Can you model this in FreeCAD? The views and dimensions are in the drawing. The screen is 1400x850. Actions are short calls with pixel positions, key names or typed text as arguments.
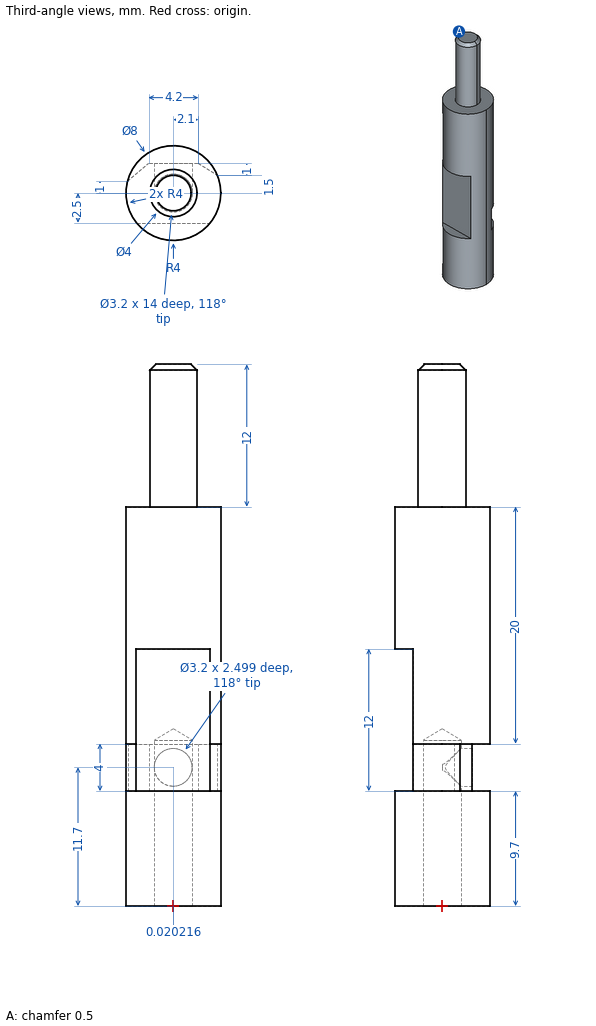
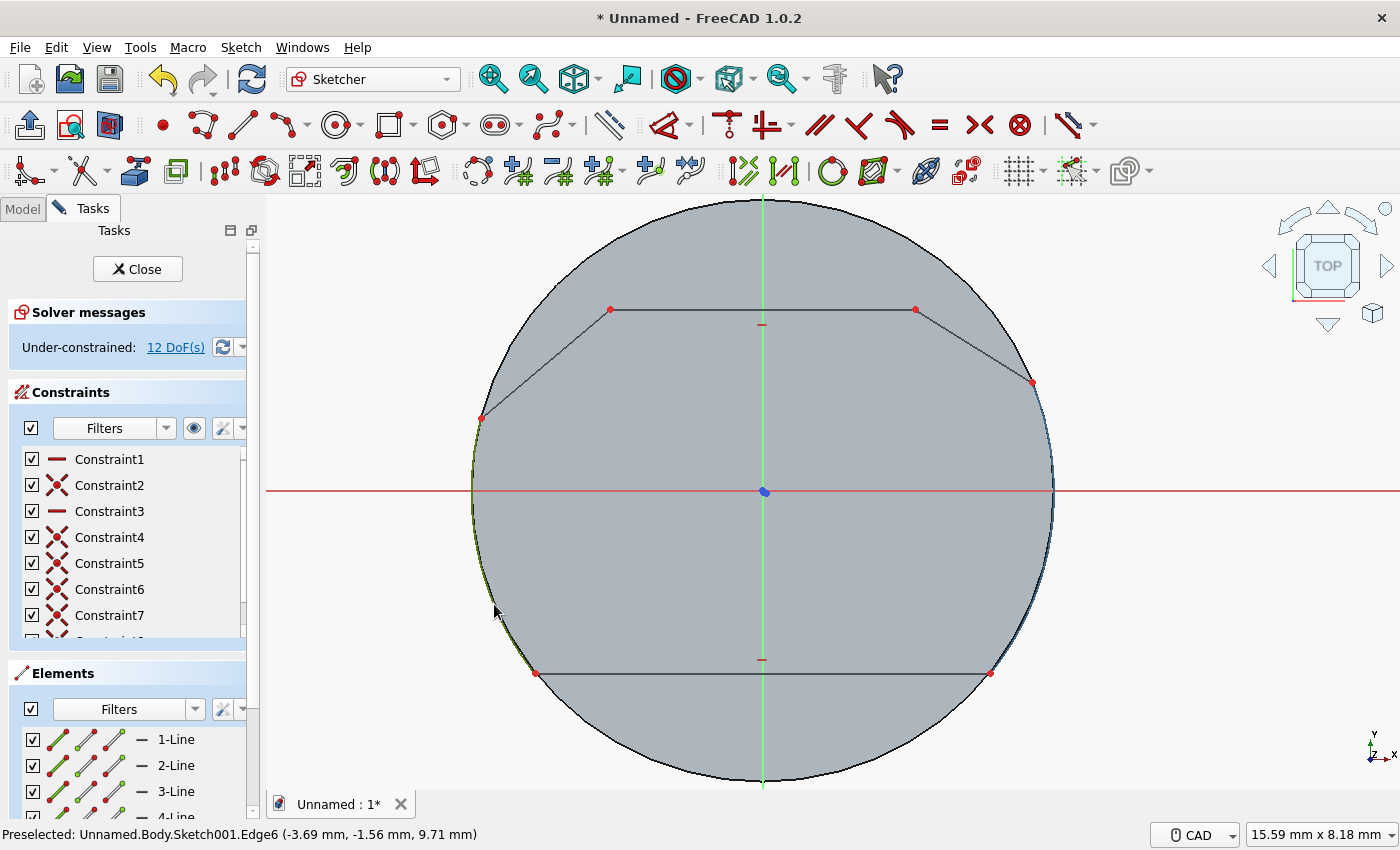
key(c)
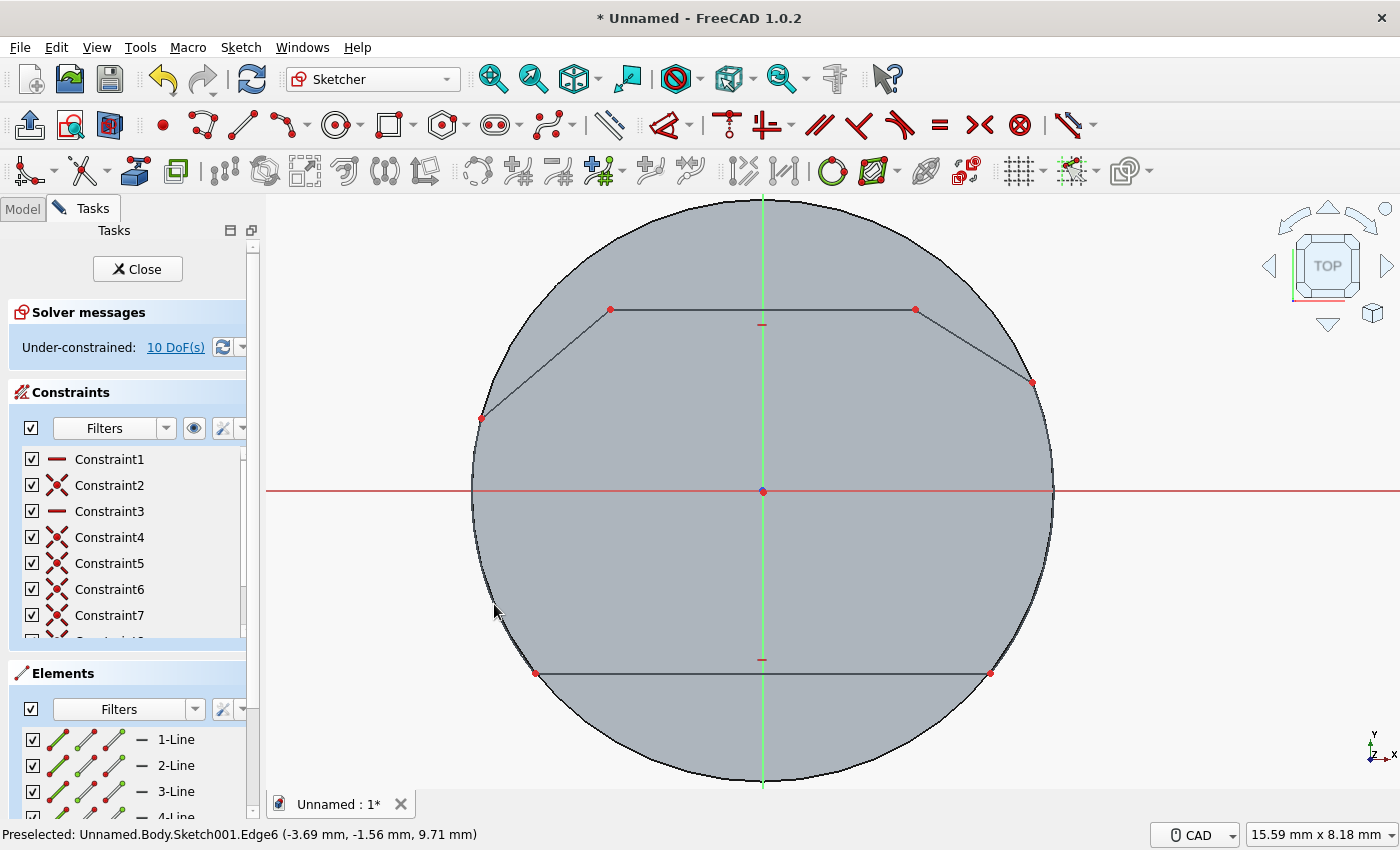
drag(753, 481, 774, 503)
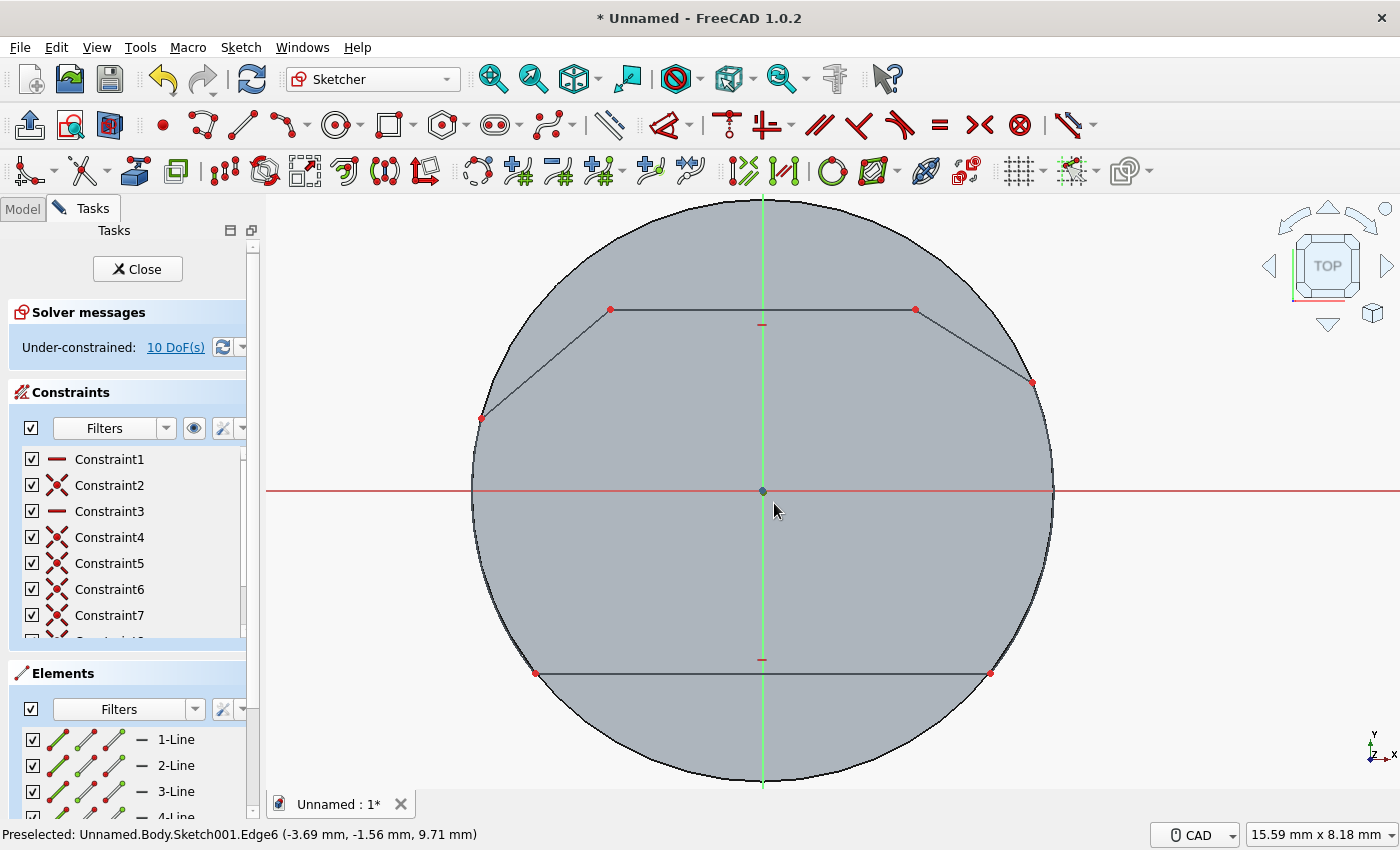
key(c)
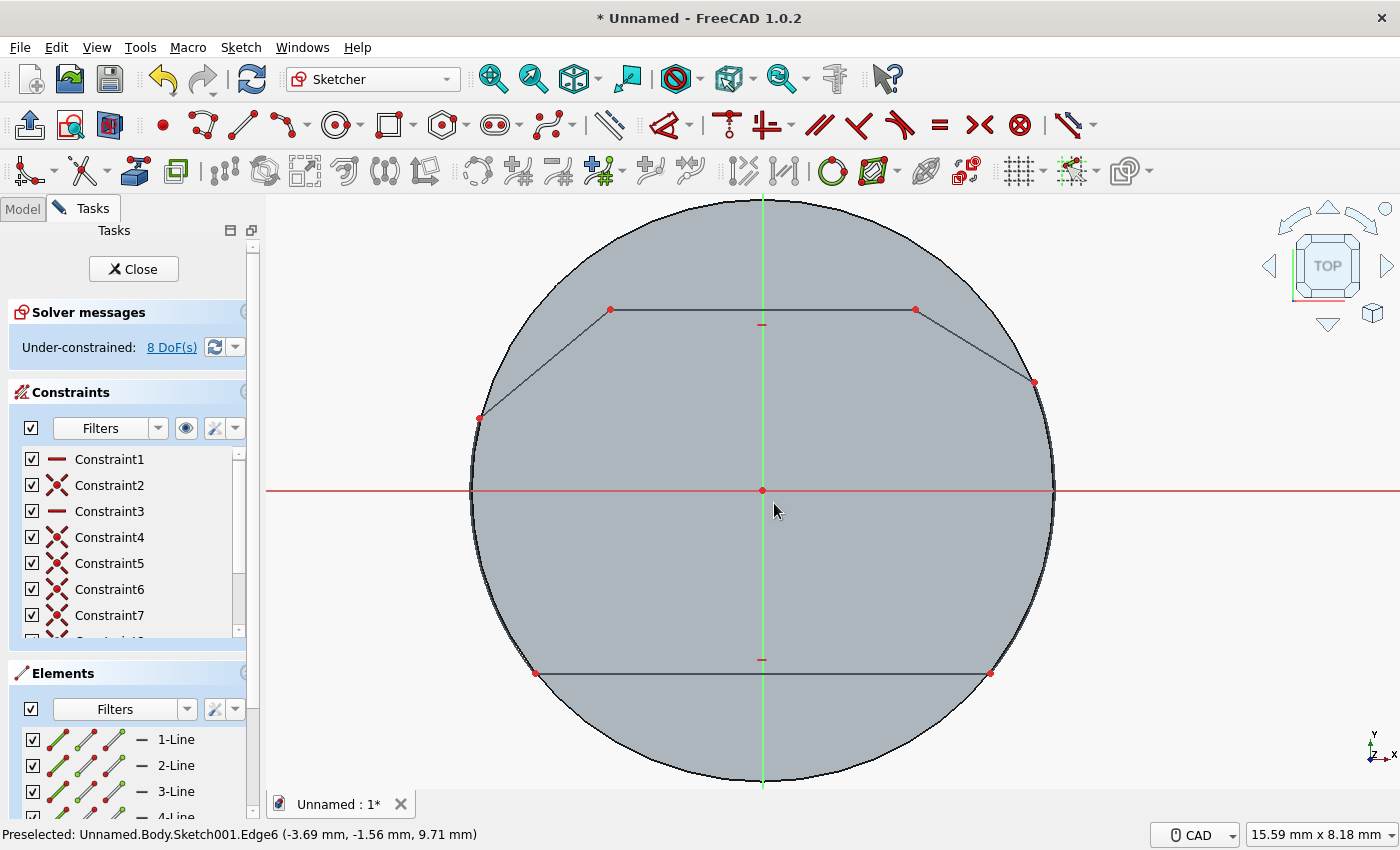
click(1036, 594)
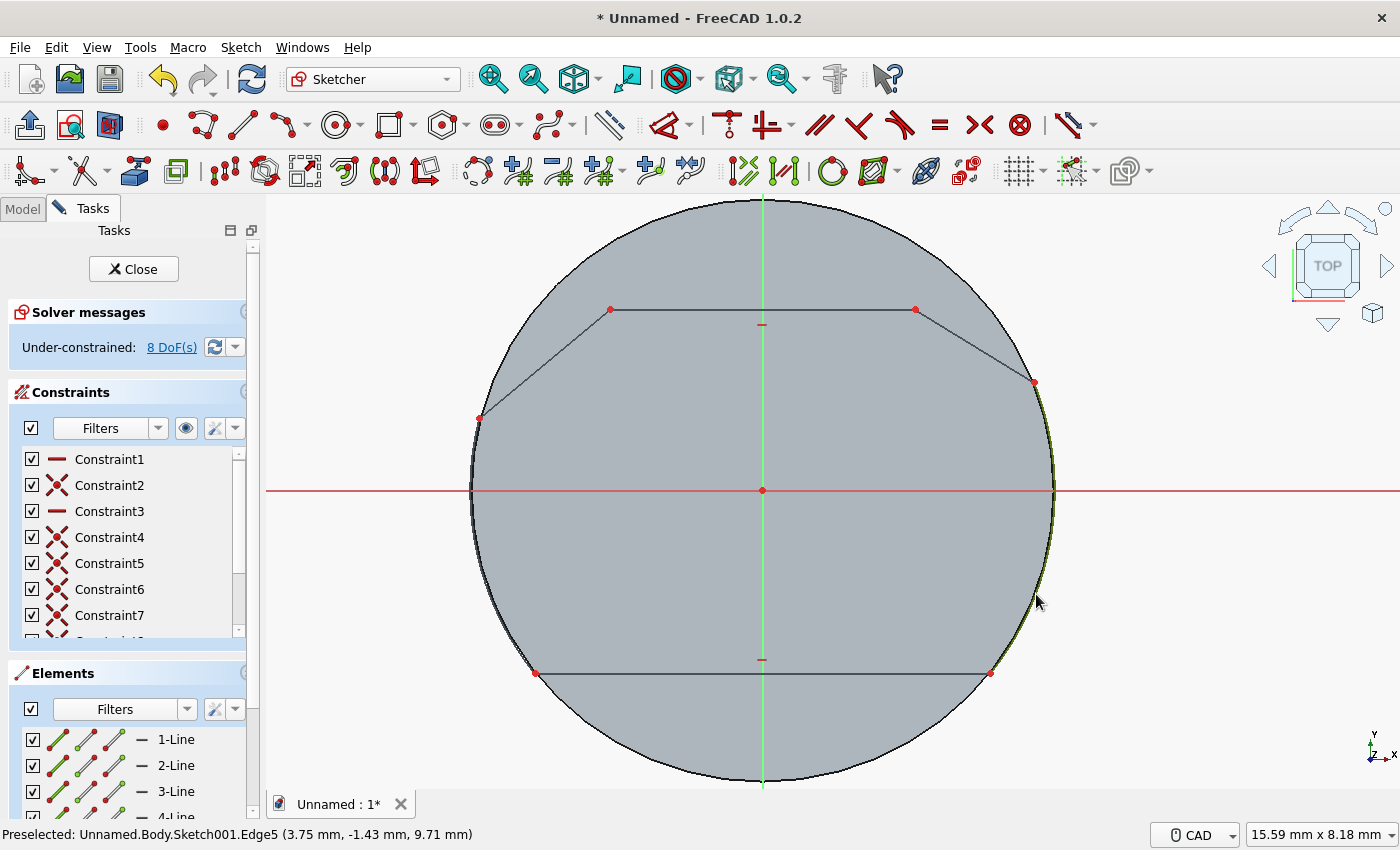
click(493, 605)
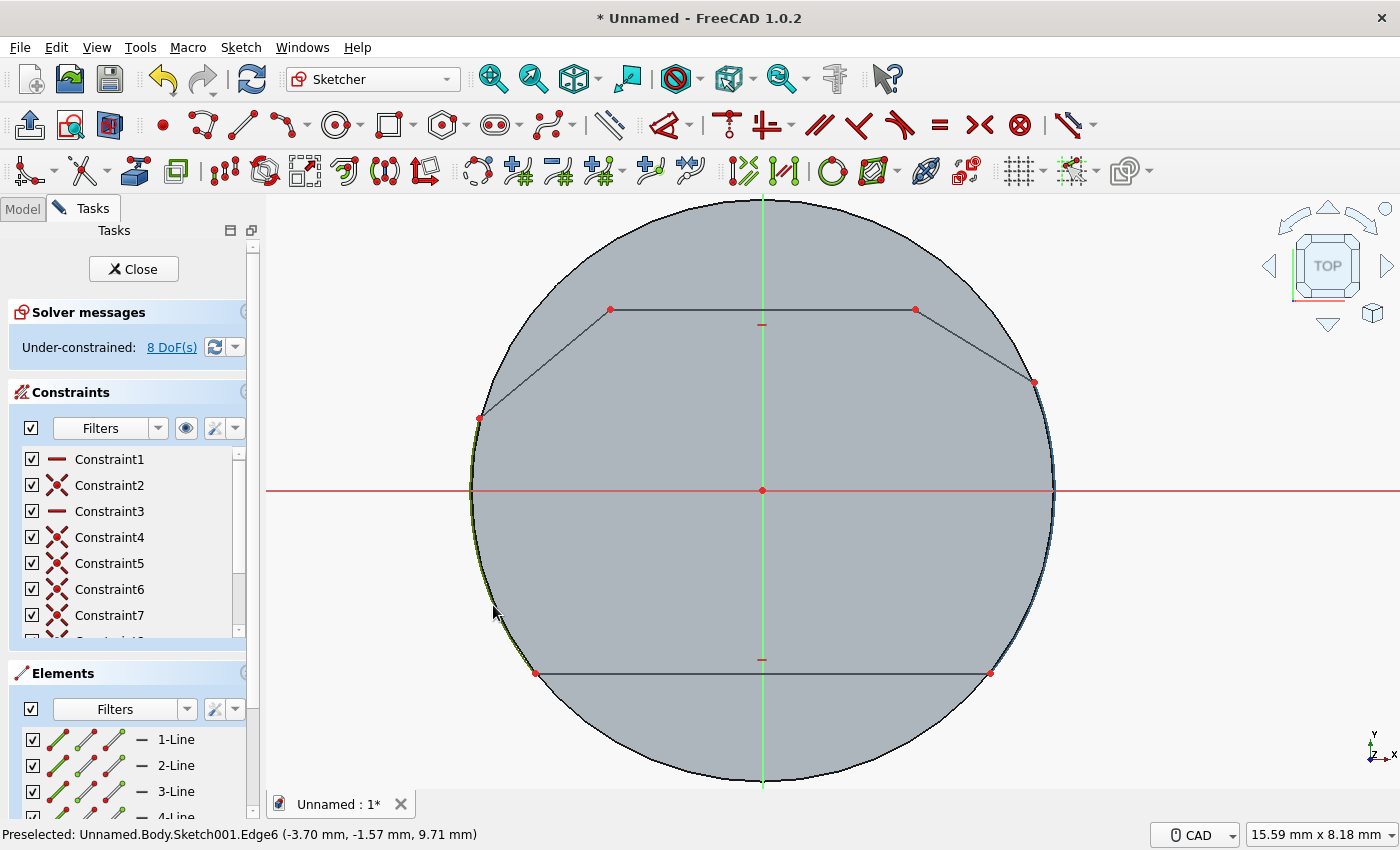
key(e)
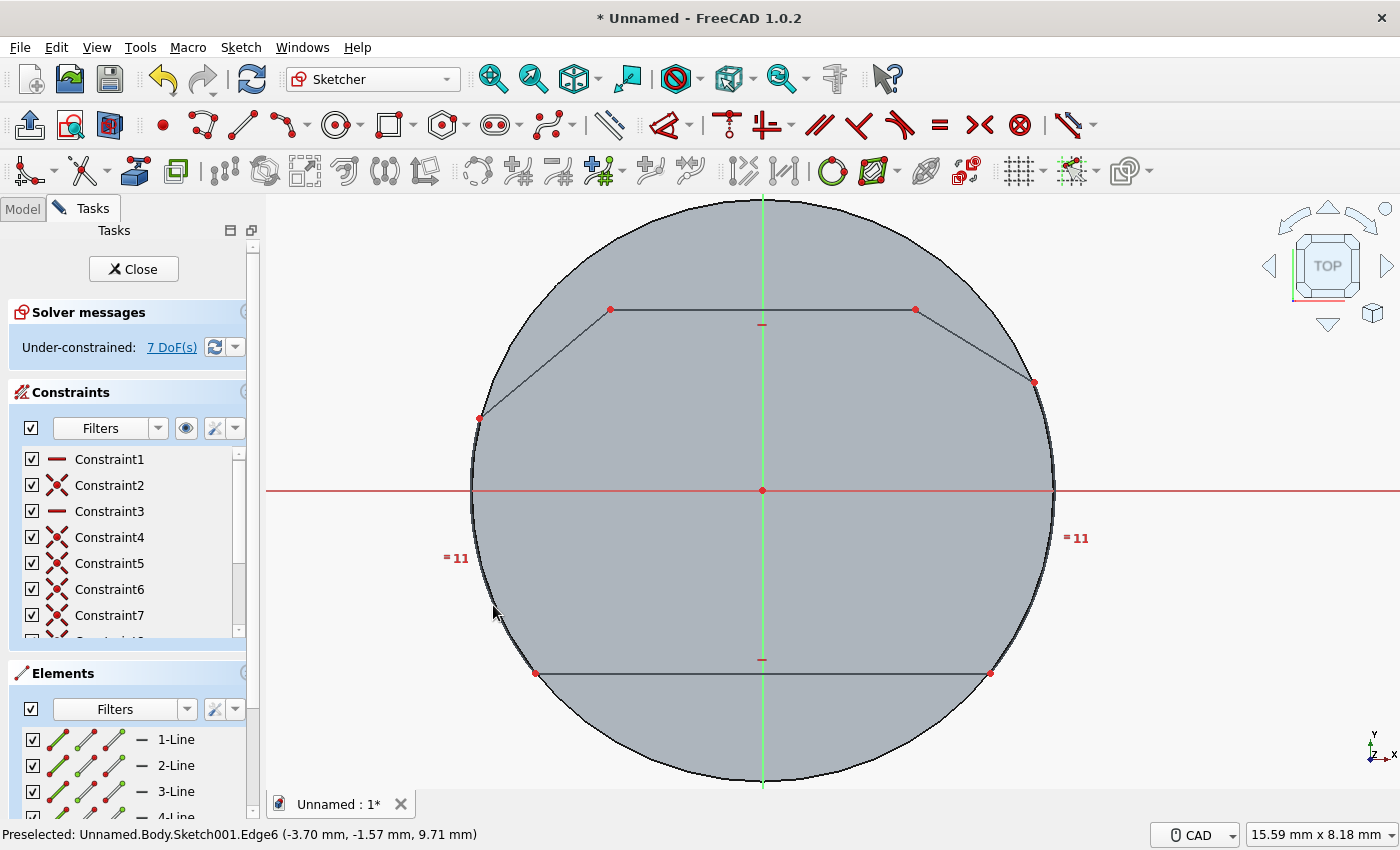
key(d)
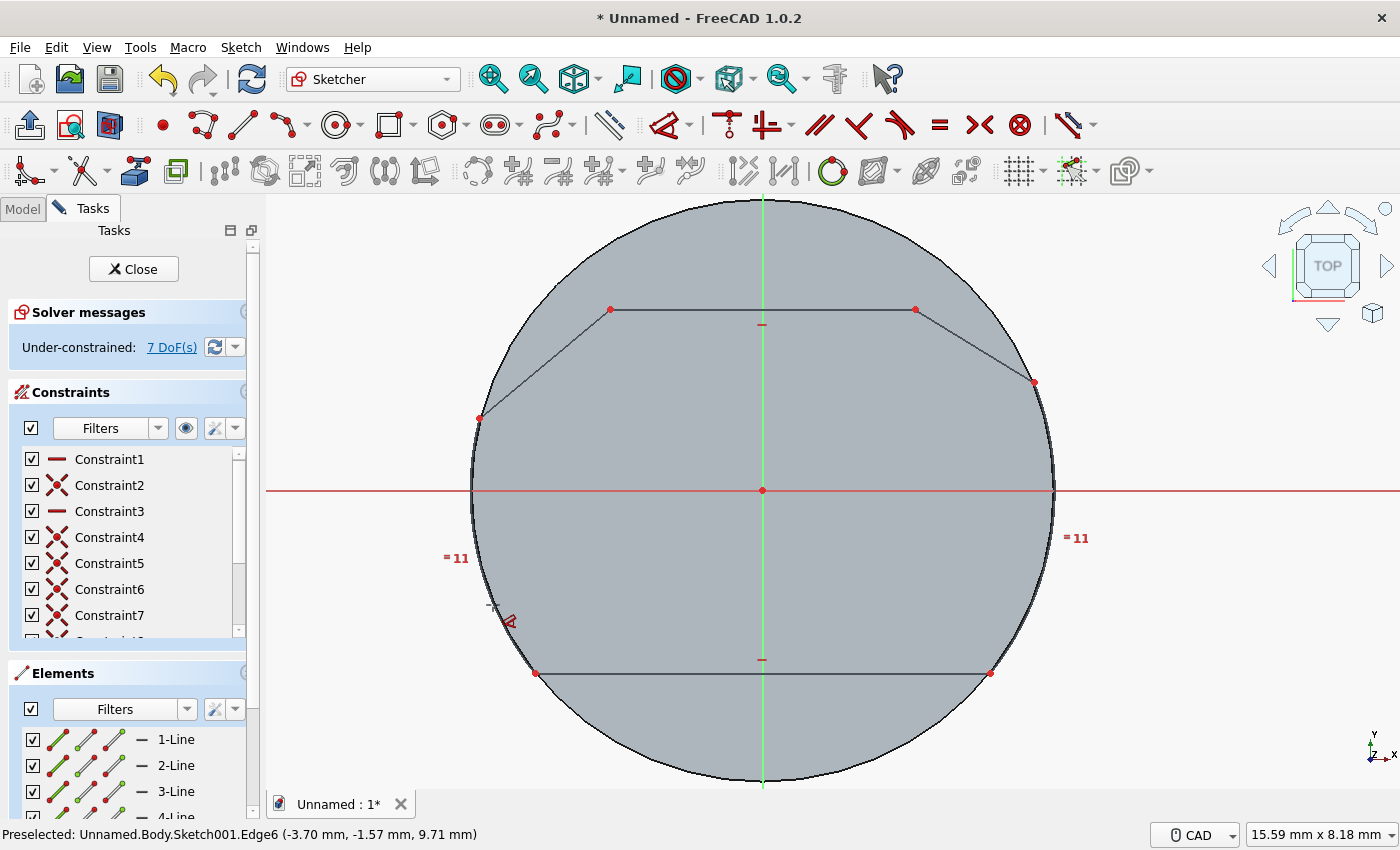
click(1036, 594)
click(1066, 605)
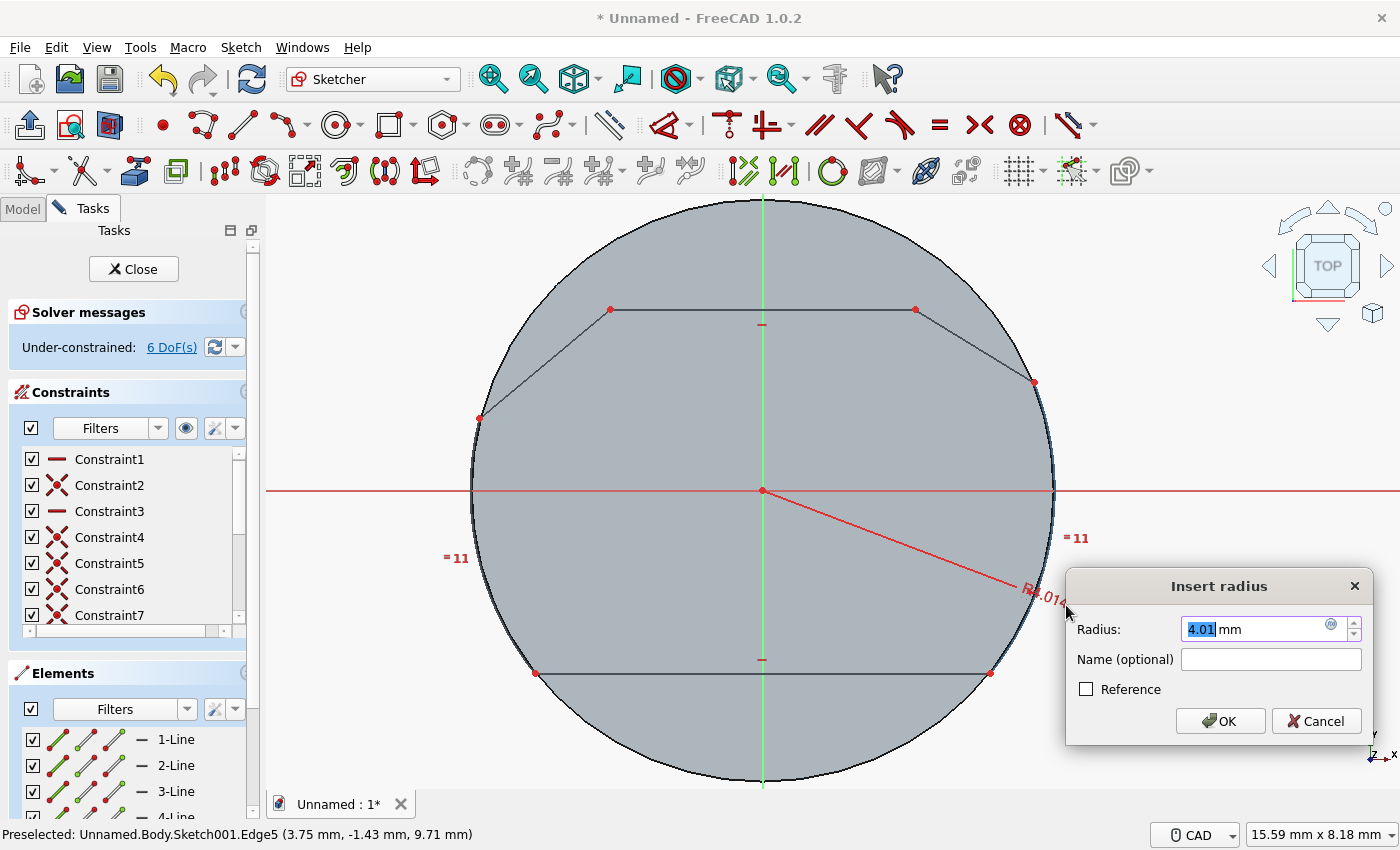
text(4)
key(Return)